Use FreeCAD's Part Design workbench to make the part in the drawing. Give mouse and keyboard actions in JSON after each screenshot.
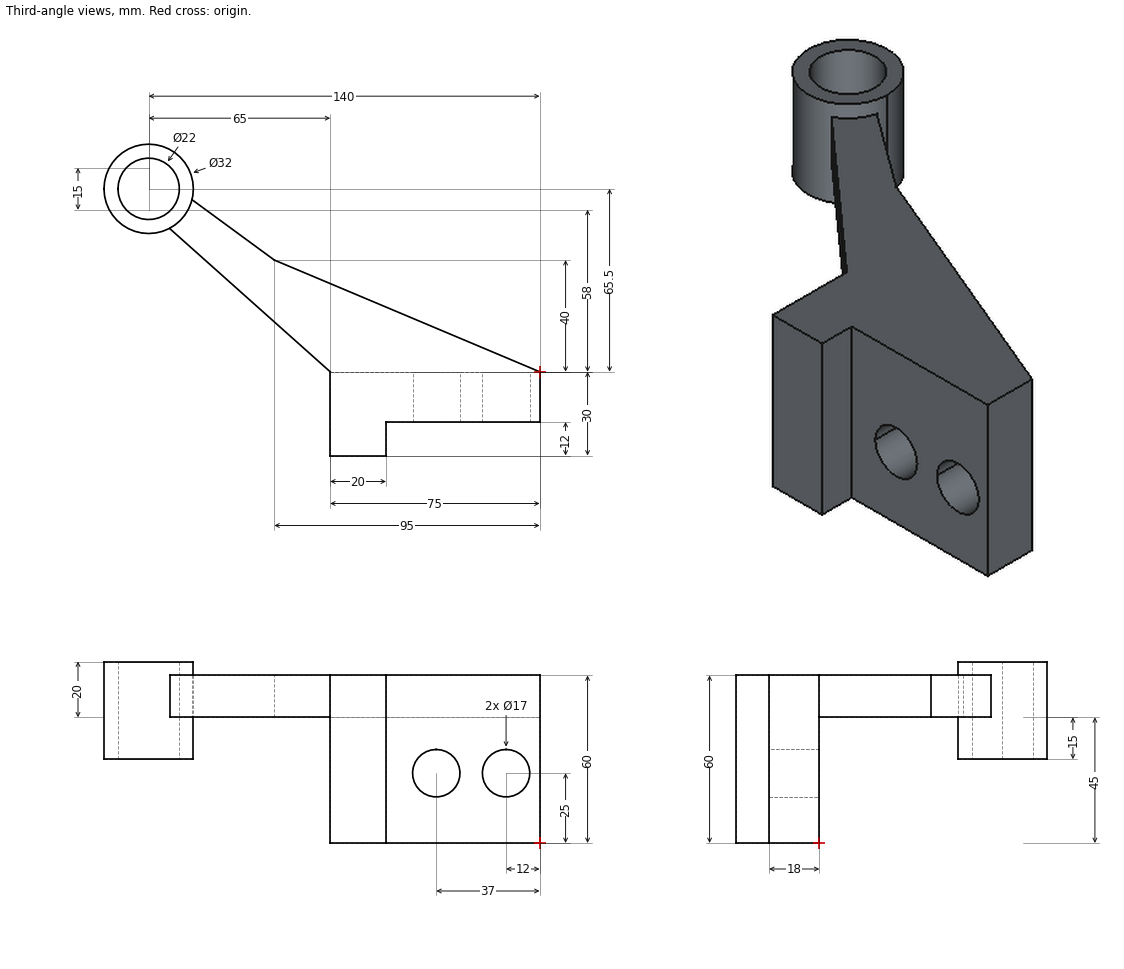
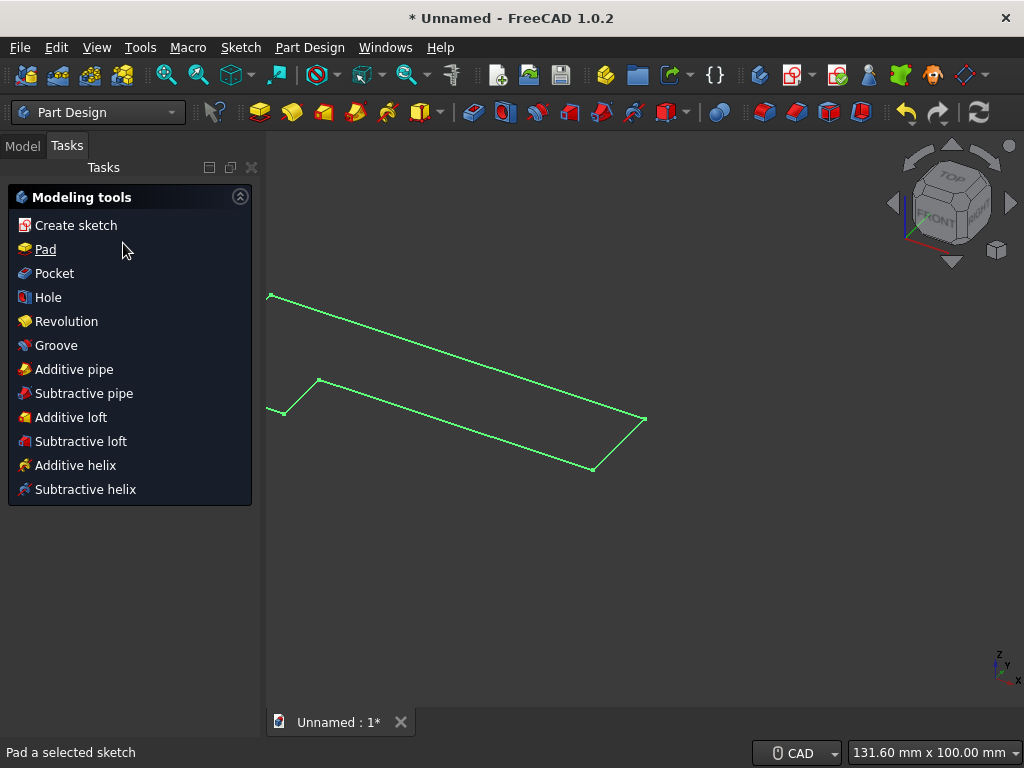
{"action": "left_click", "coordinate": [260, 112]}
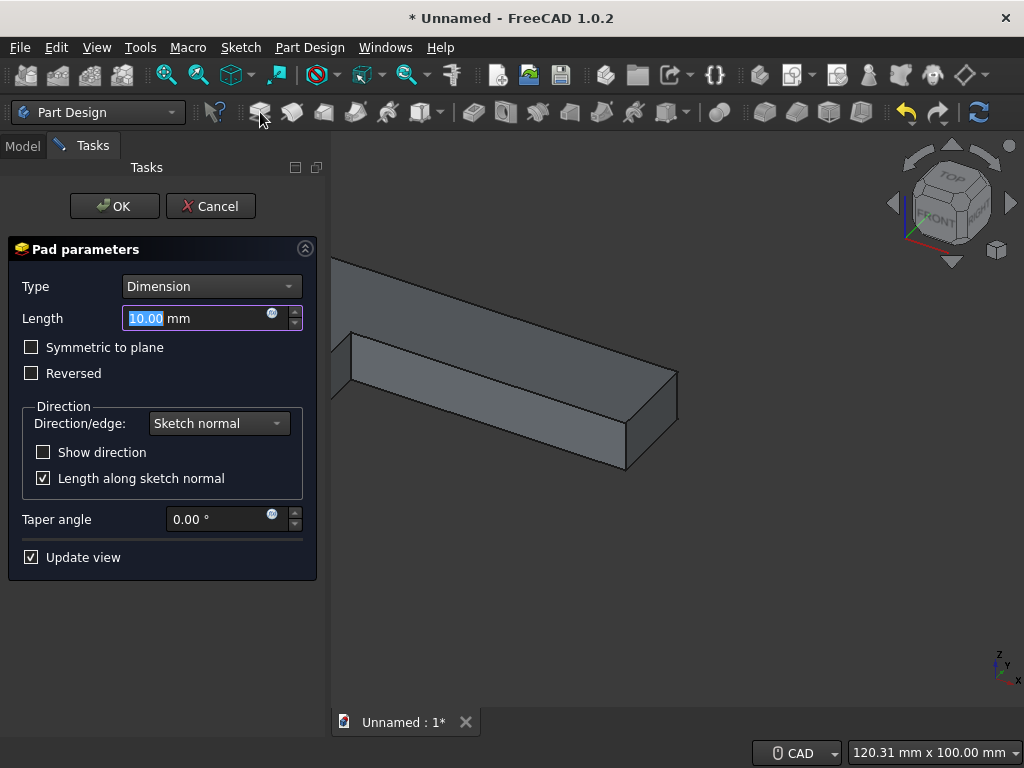
{"action": "type", "text": "60"}
{"action": "key", "text": "Tab"}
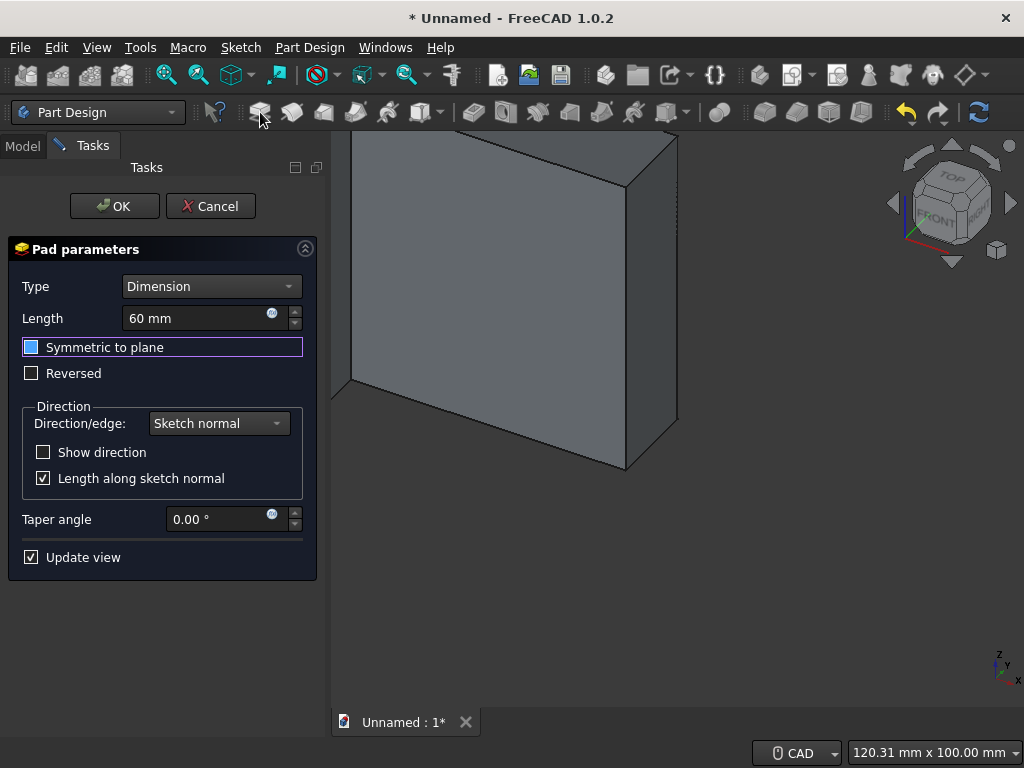
{"action": "left_click", "coordinate": [115, 206]}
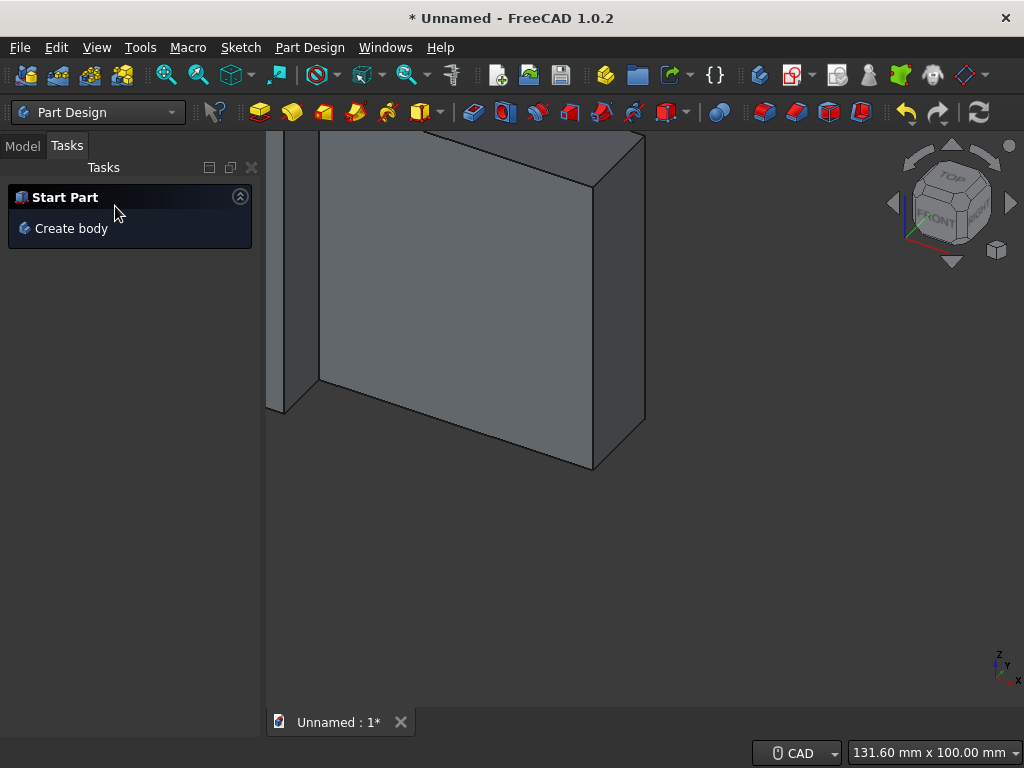
{"action": "left_click", "coordinate": [168, 76]}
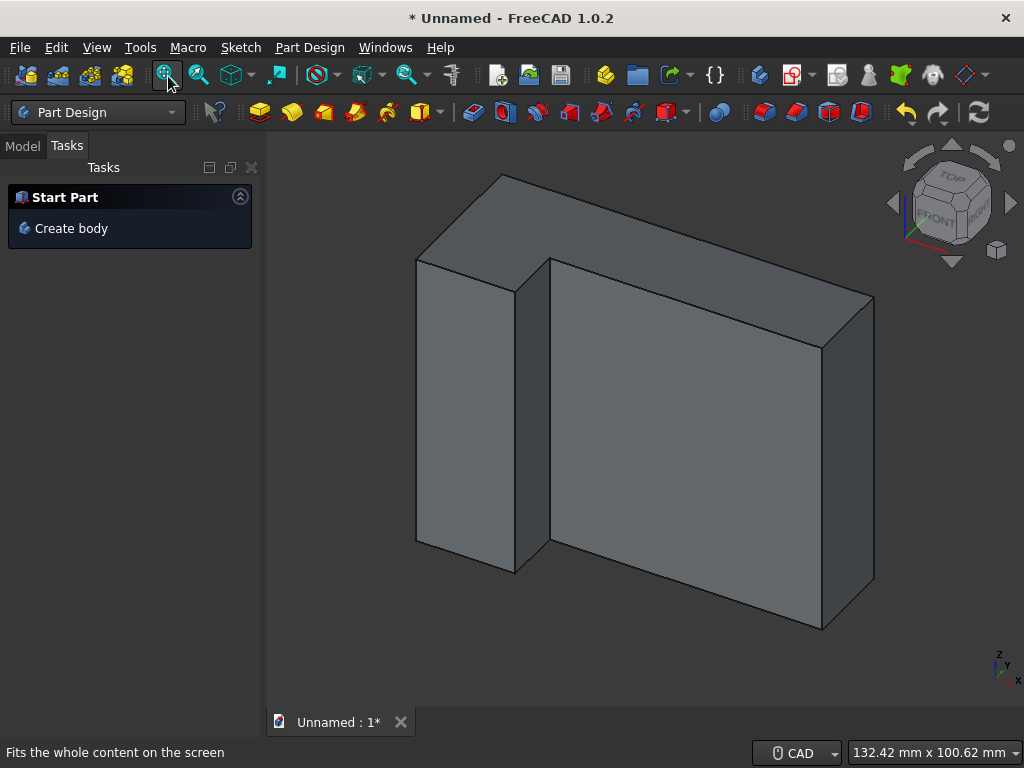
{"action": "key", "text": "5"}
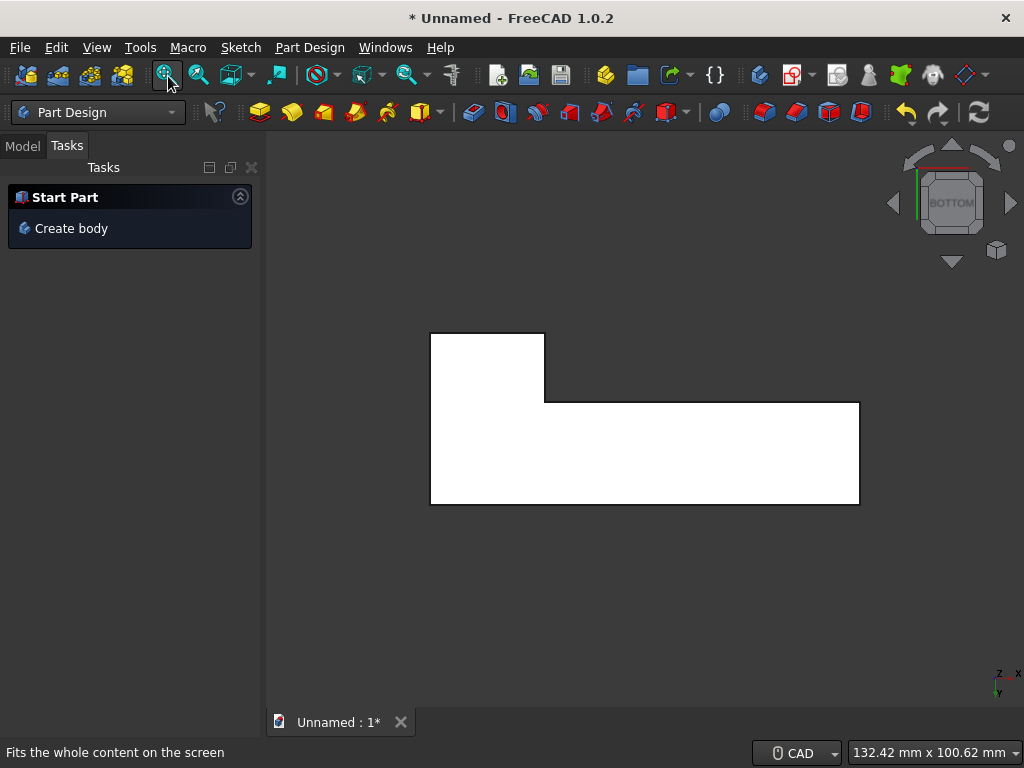
{"action": "left_click", "coordinate": [522, 443]}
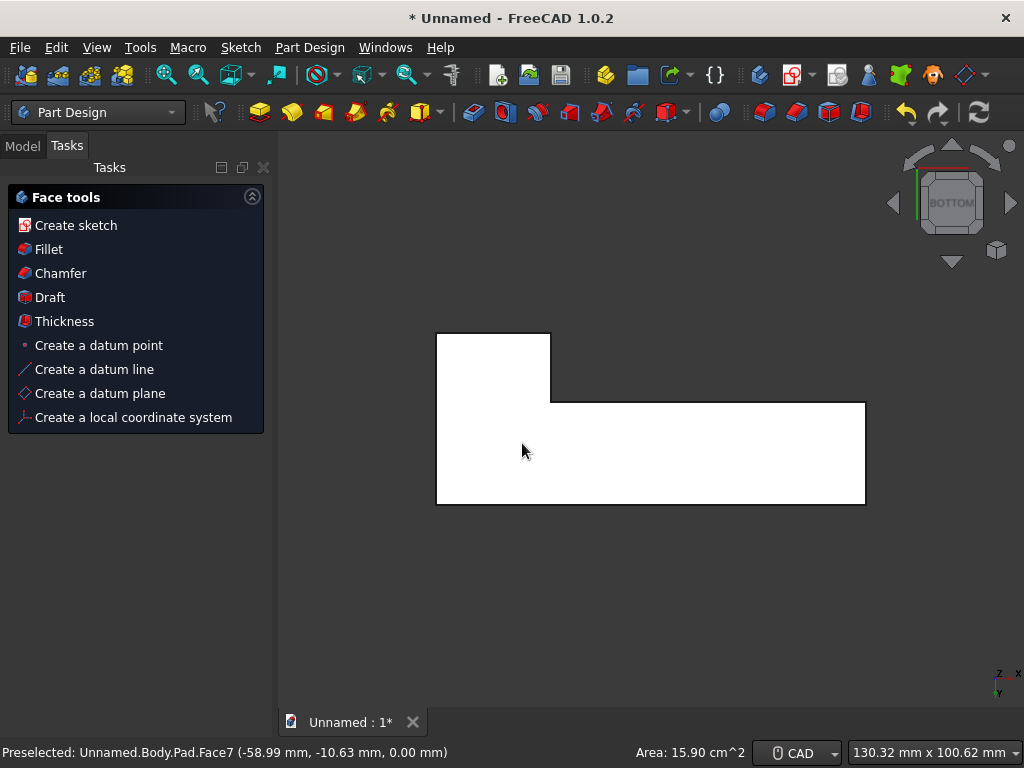
{"action": "left_click", "coordinate": [792, 76]}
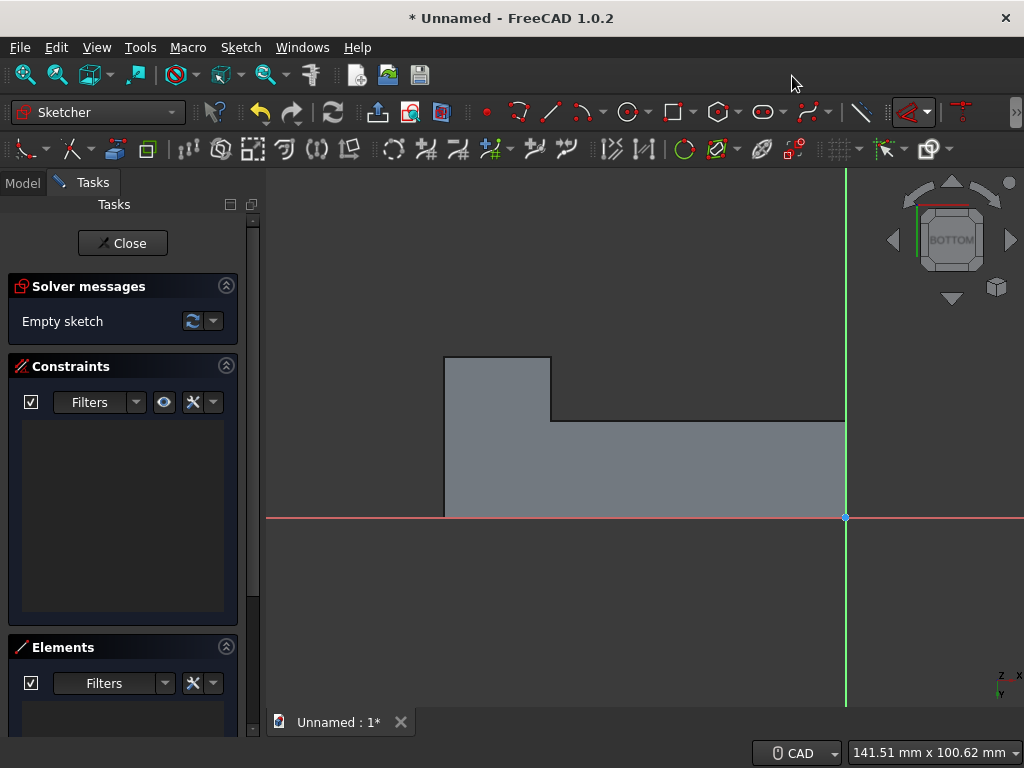
{"action": "scroll", "coordinate": [705, 196], "scroll_direction": "down", "scroll_amount": 3}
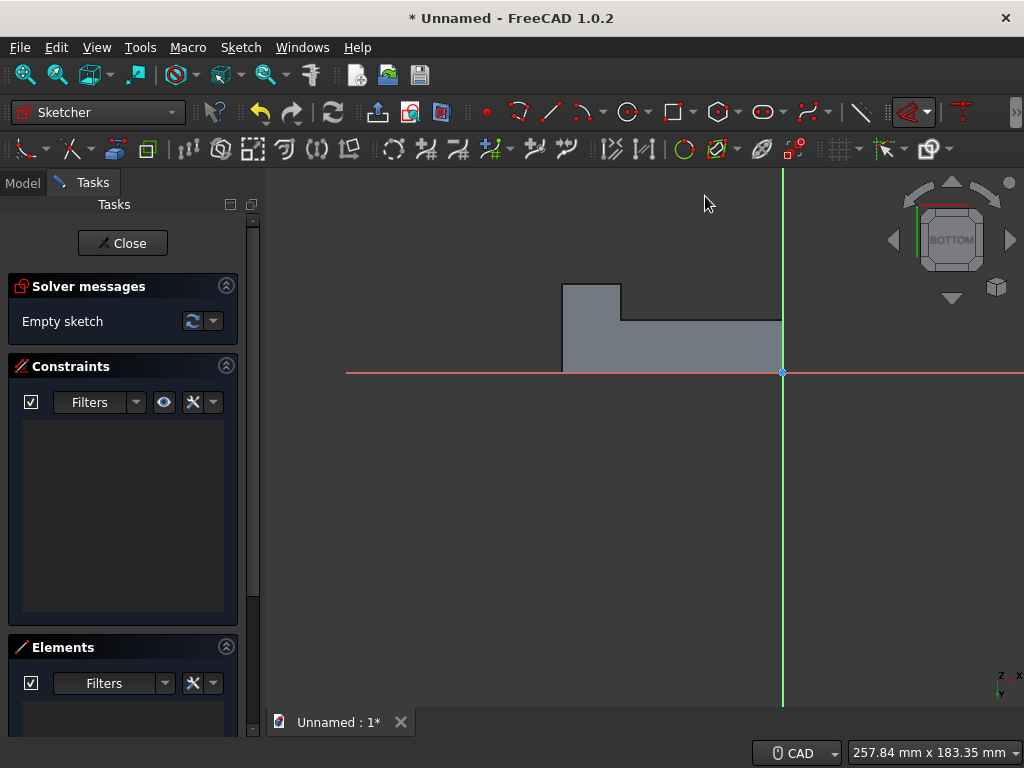
{"action": "left_click", "coordinate": [520, 112]}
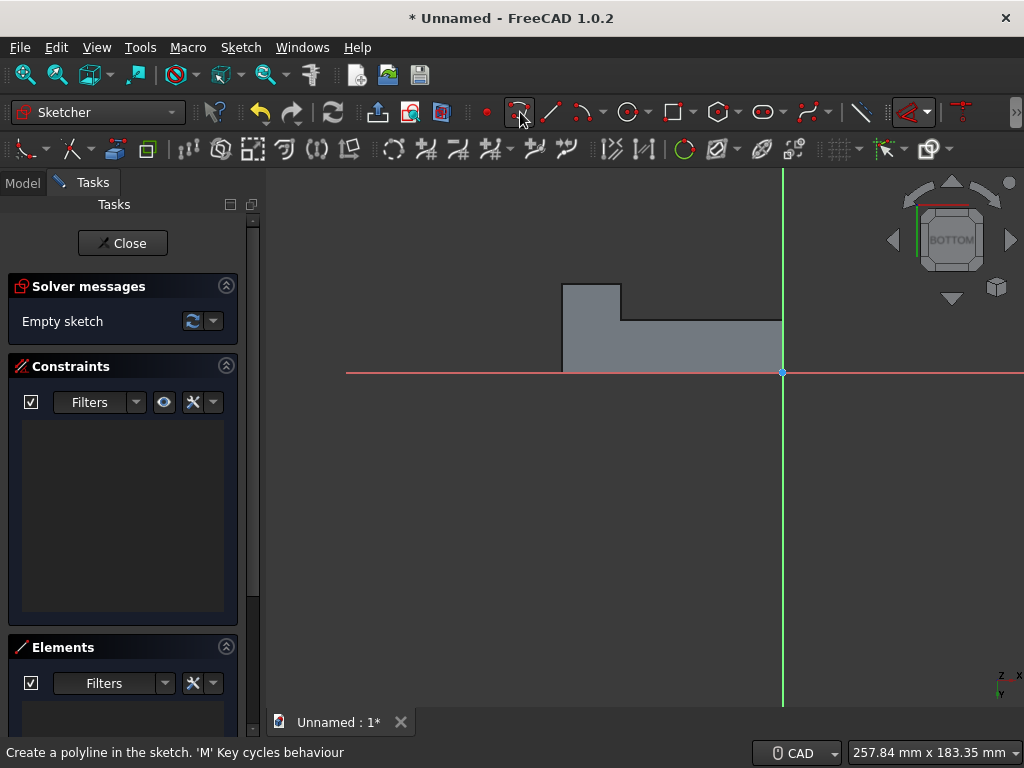
{"action": "left_click", "coordinate": [783, 373]}
{"action": "left_click", "coordinate": [562, 382]}
{"action": "left_click", "coordinate": [371, 543]}
{"action": "left_click", "coordinate": [371, 587]}
{"action": "left_click", "coordinate": [503, 490]}
{"action": "left_click", "coordinate": [783, 373]}
{"action": "key", "text": "Escape"}
{"action": "key", "text": "Escape"}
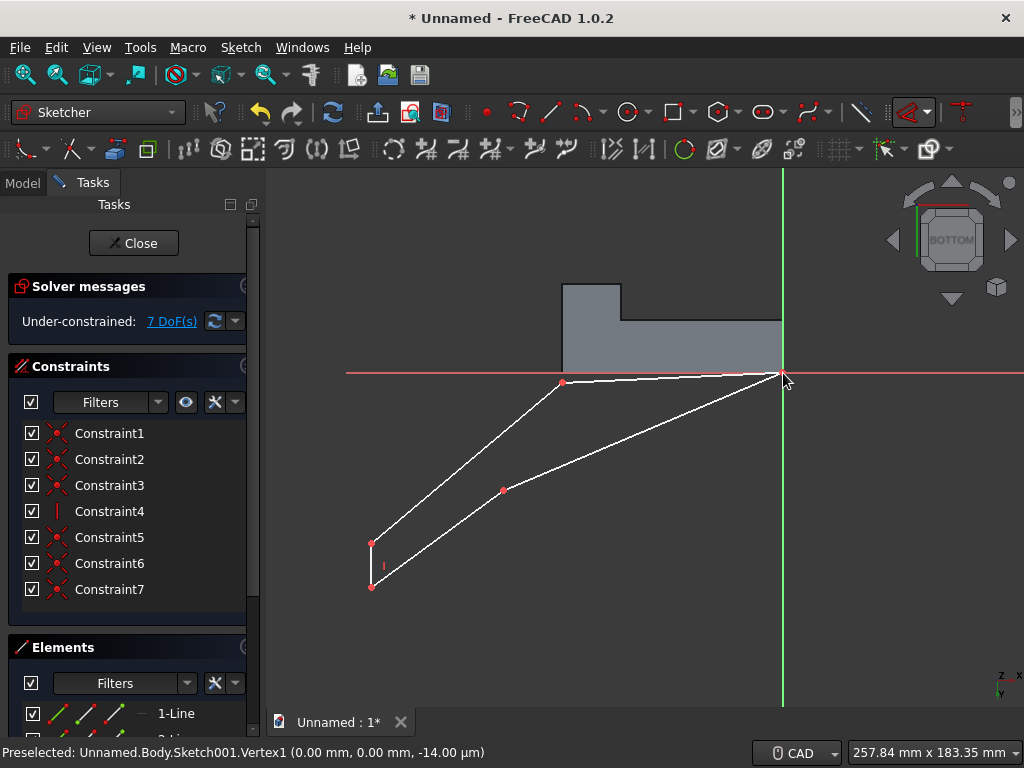
{"action": "left_click", "coordinate": [716, 376]}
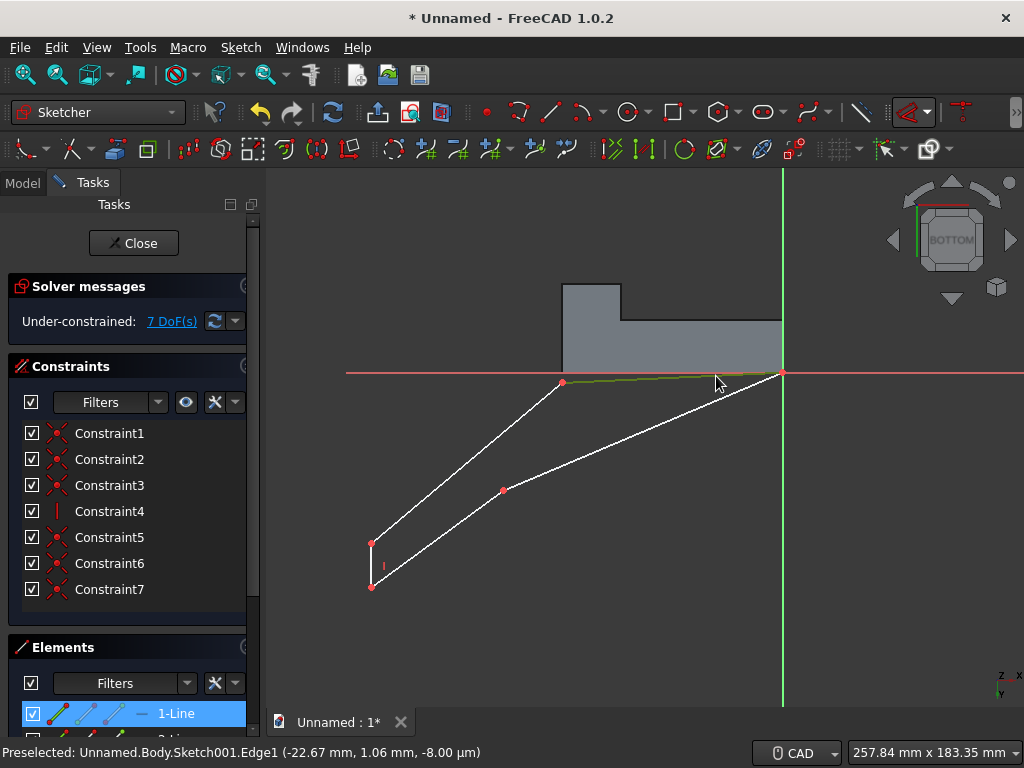
{"action": "key", "text": "h"}